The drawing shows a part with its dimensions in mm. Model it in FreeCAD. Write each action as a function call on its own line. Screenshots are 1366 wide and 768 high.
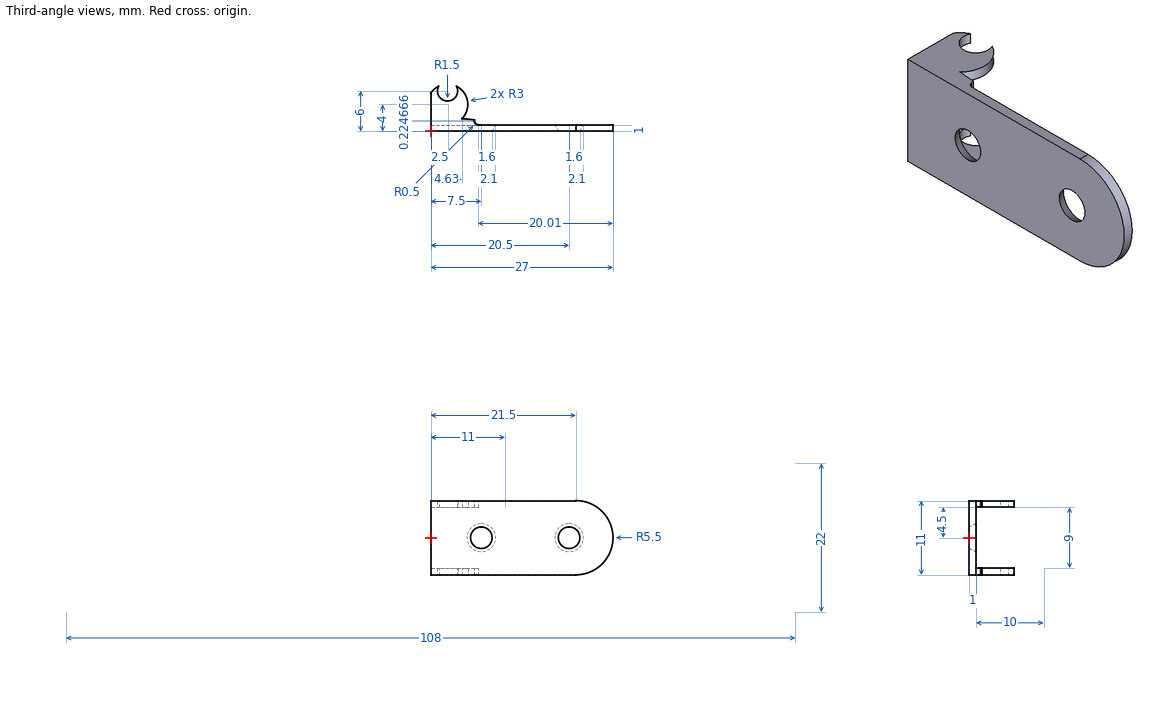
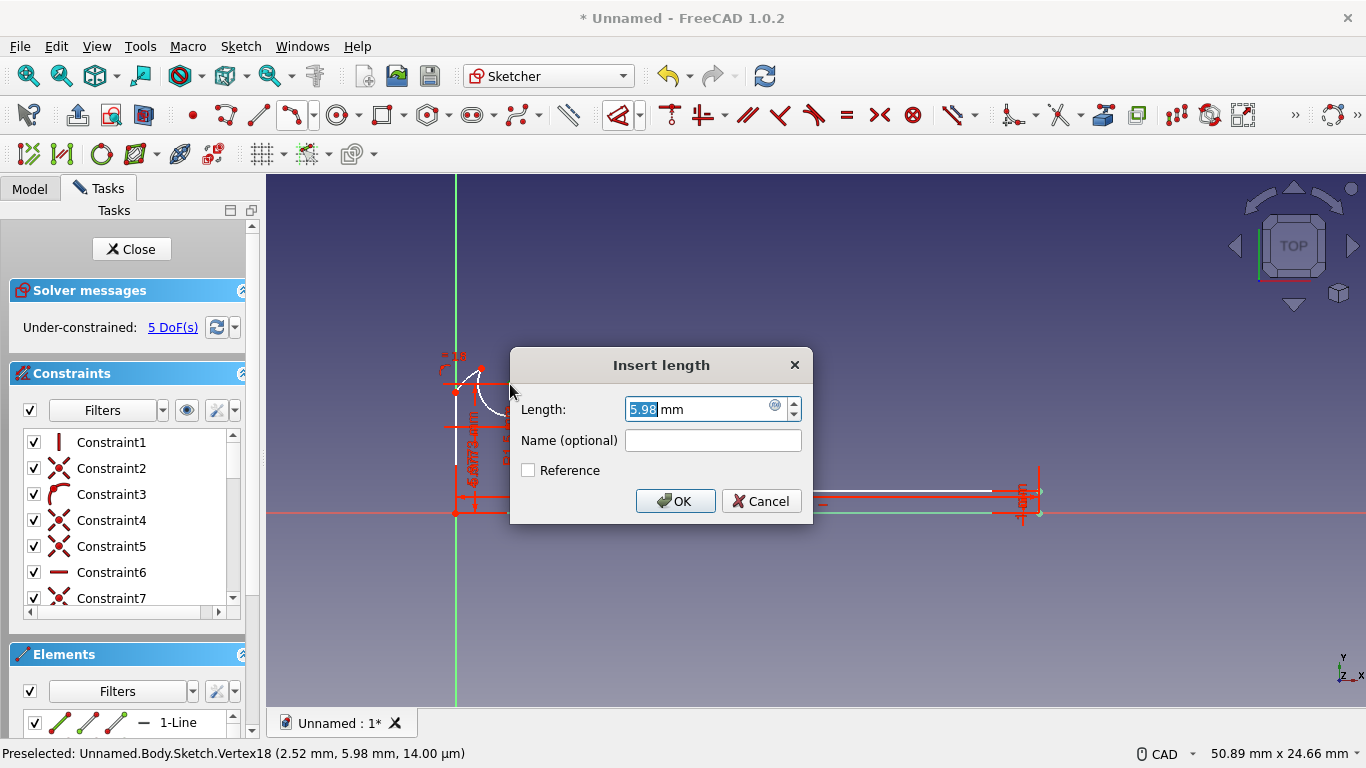
text(6)
key(Return)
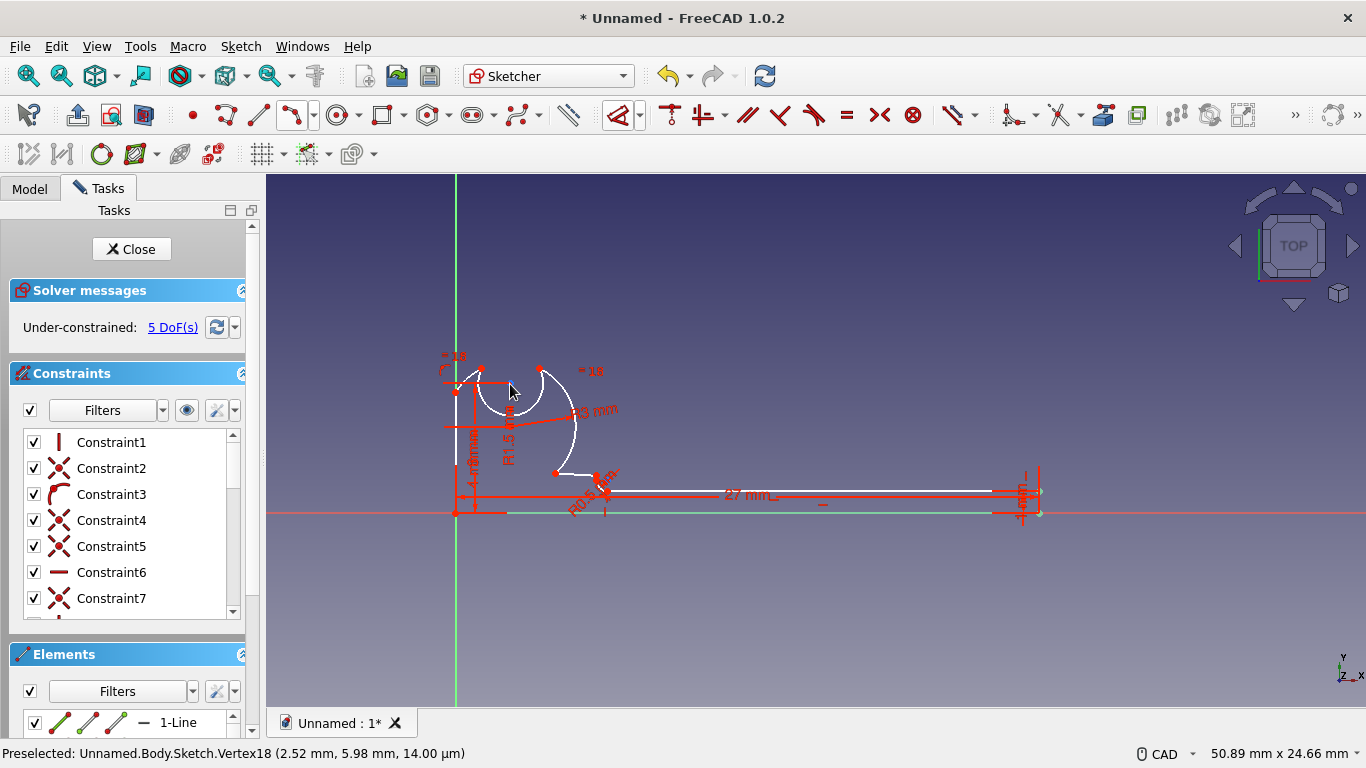
click(511, 427)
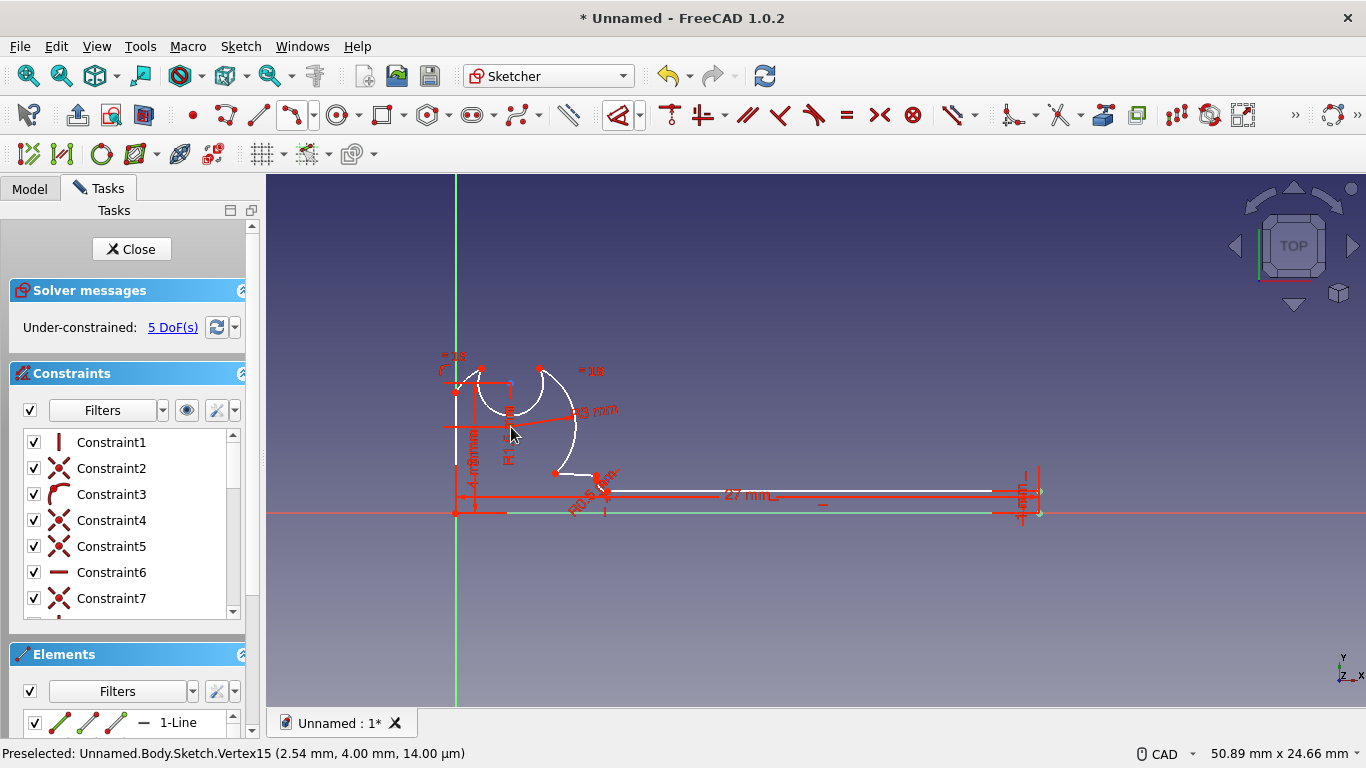
key(l)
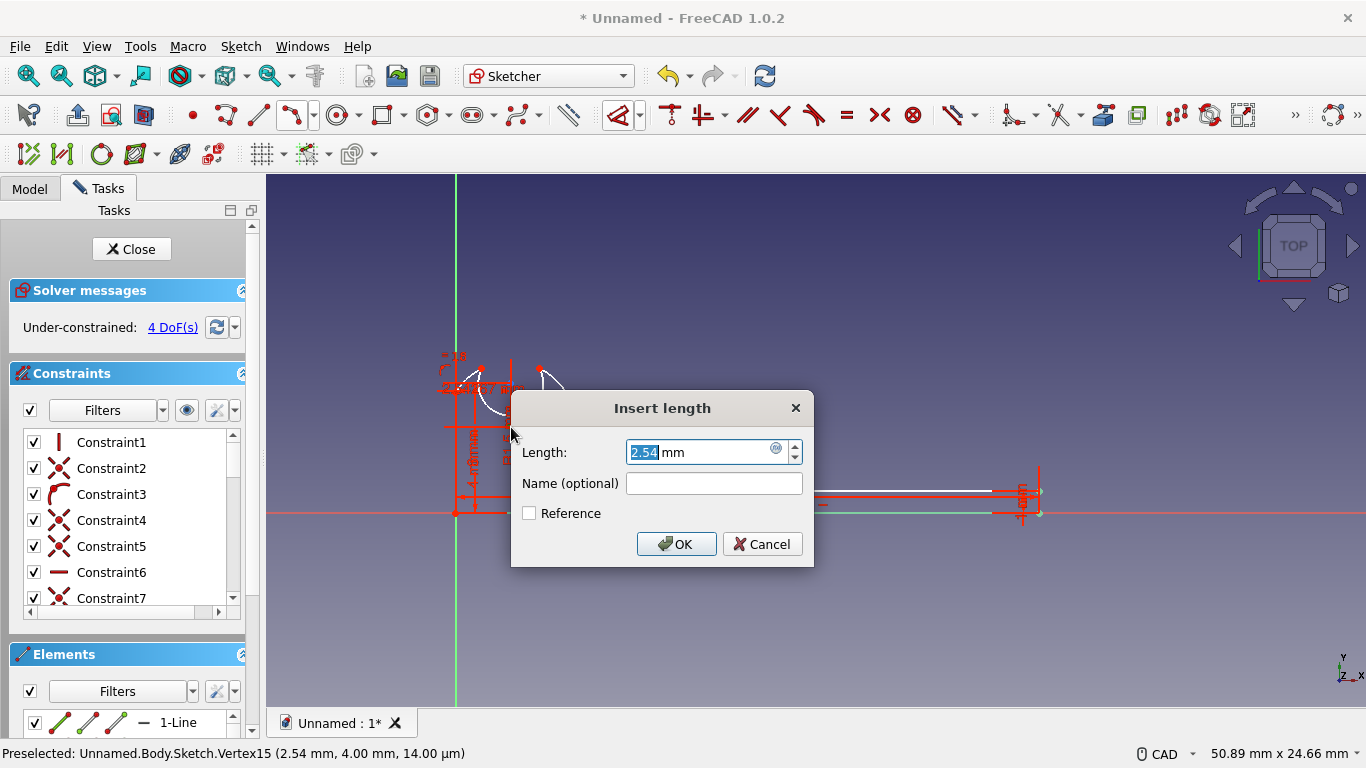
text(2.5)
key(Return)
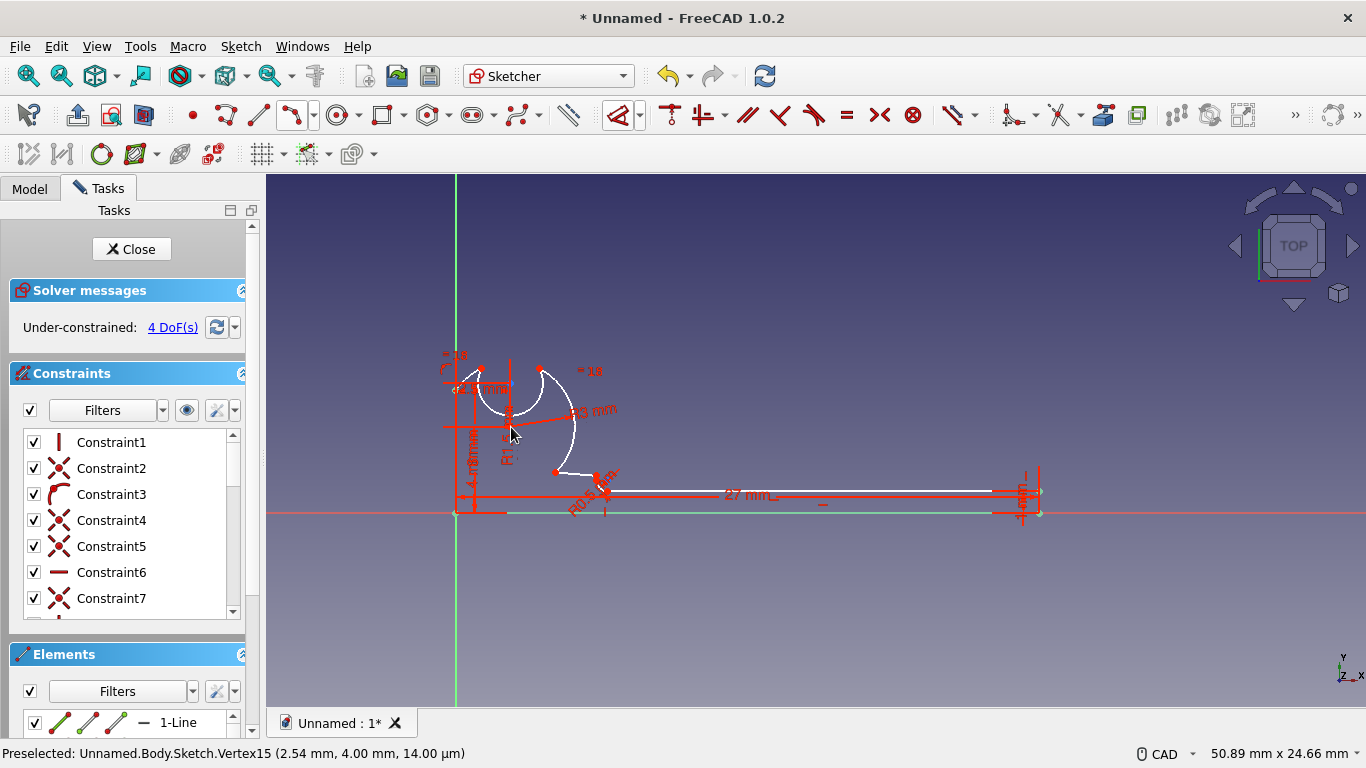
click(510, 383)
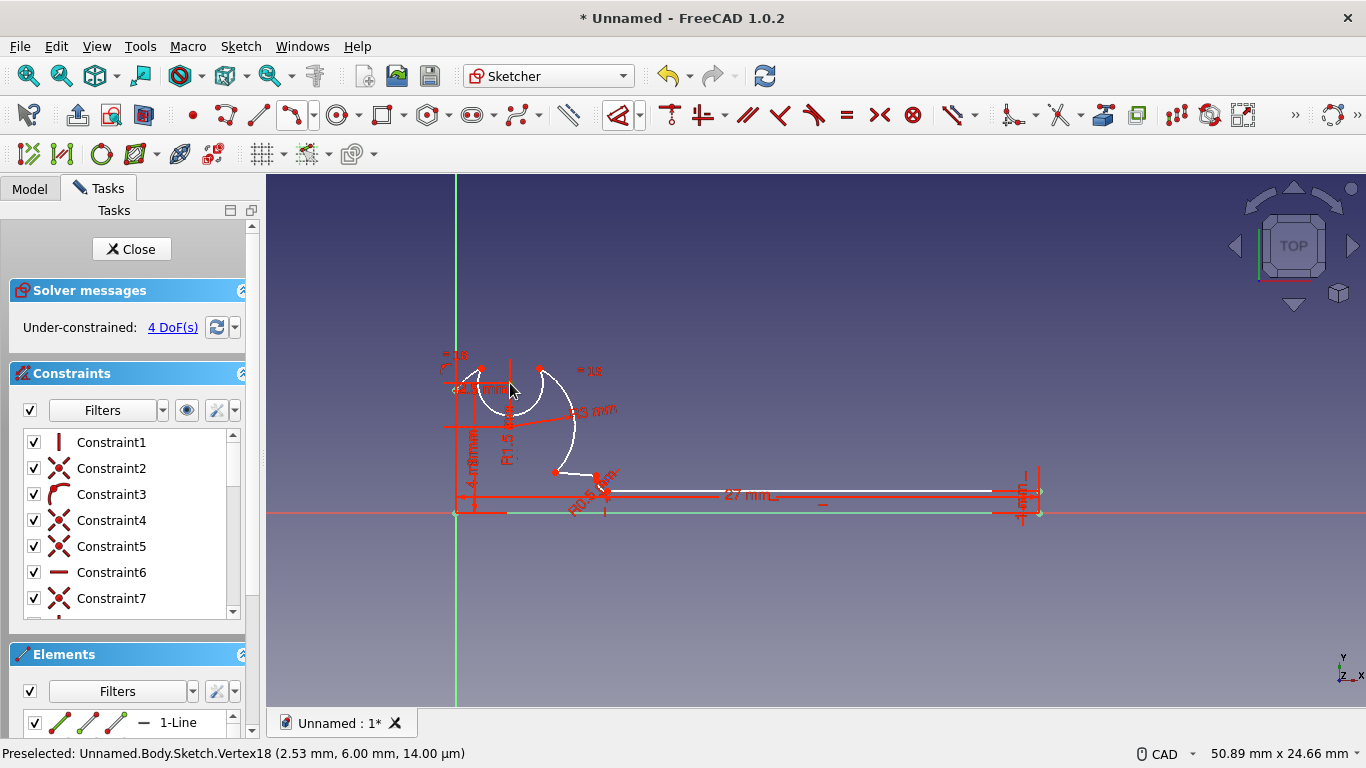
key(l)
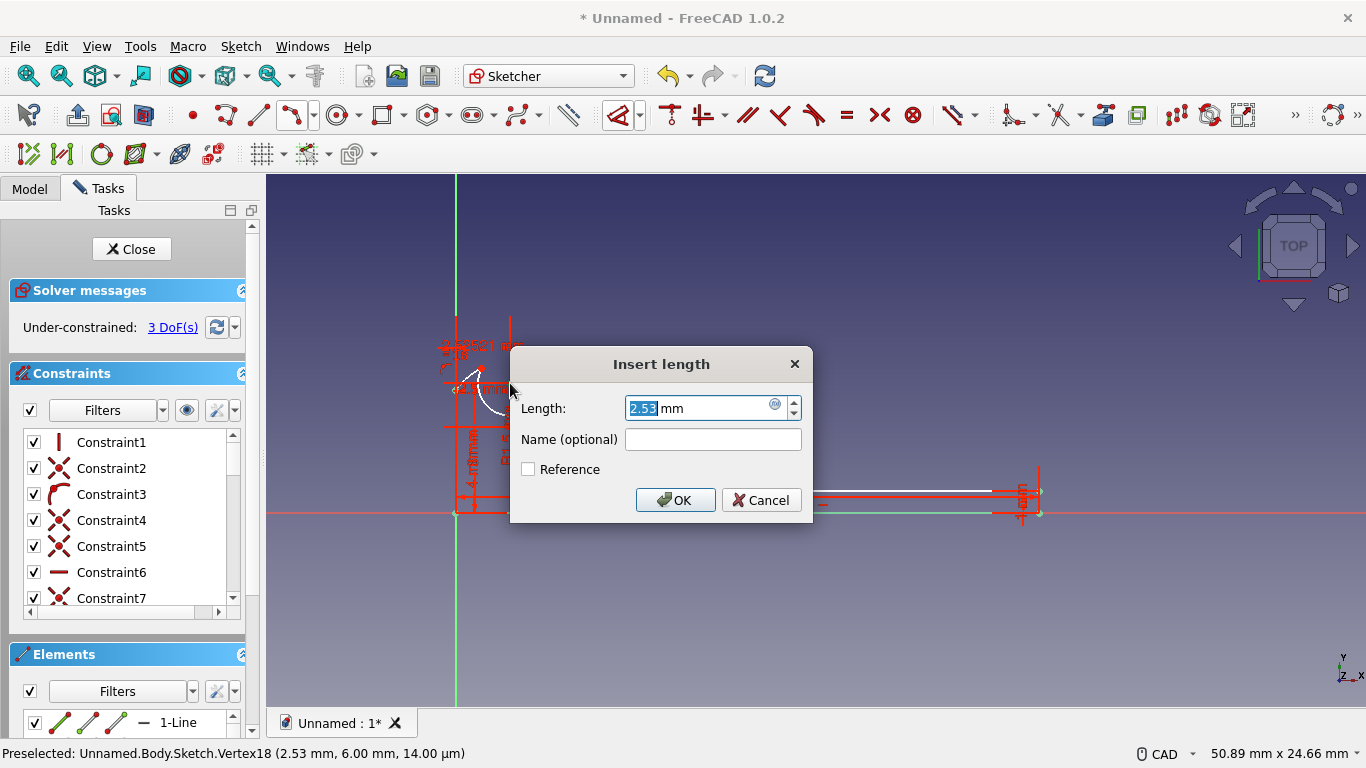
text(2.5)
key(Return)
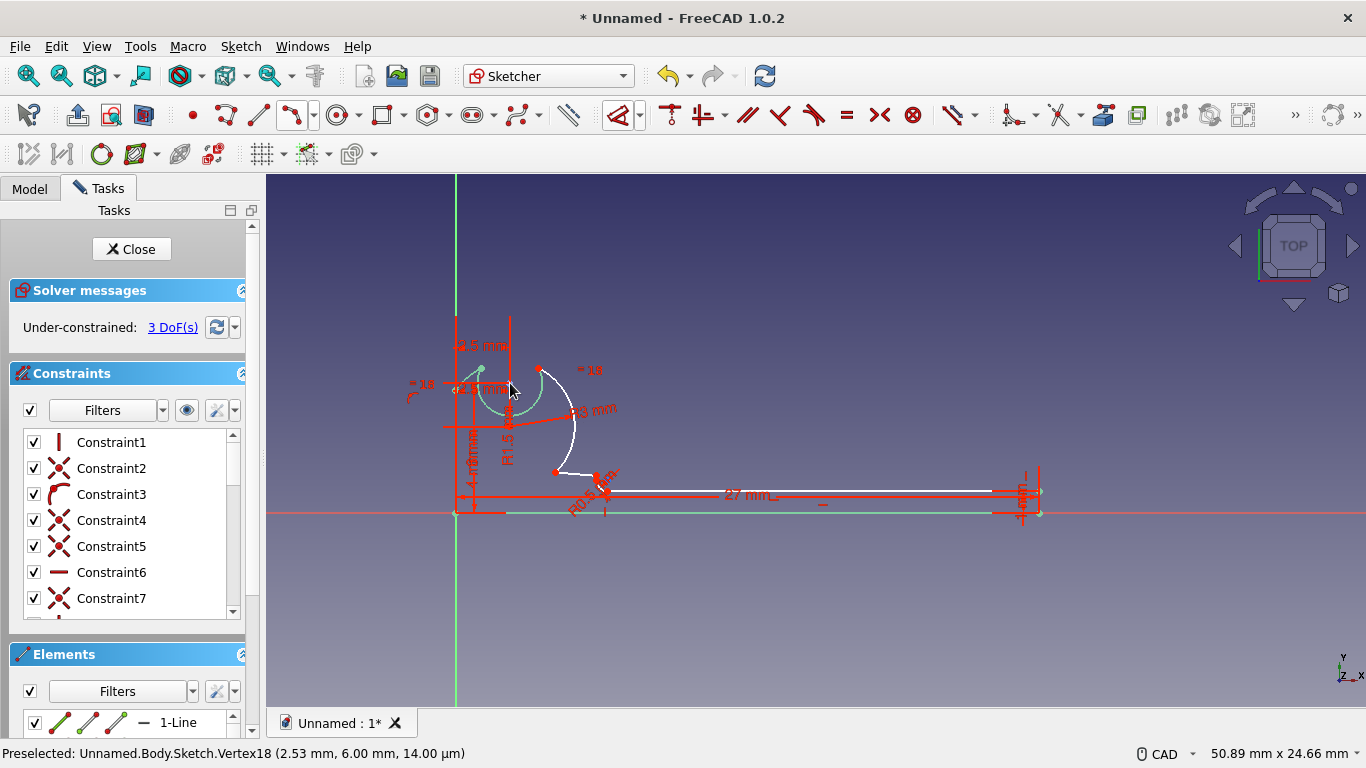
click(910, 491)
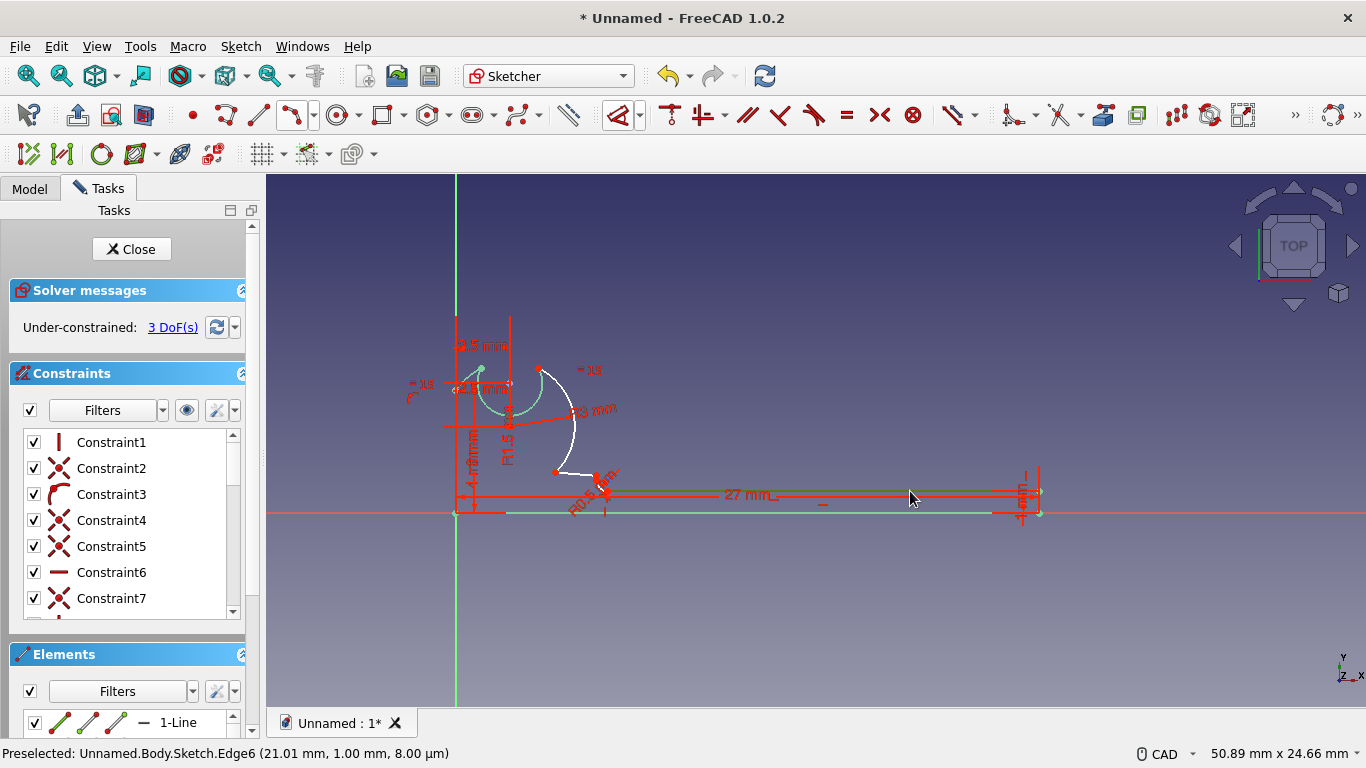
key(l)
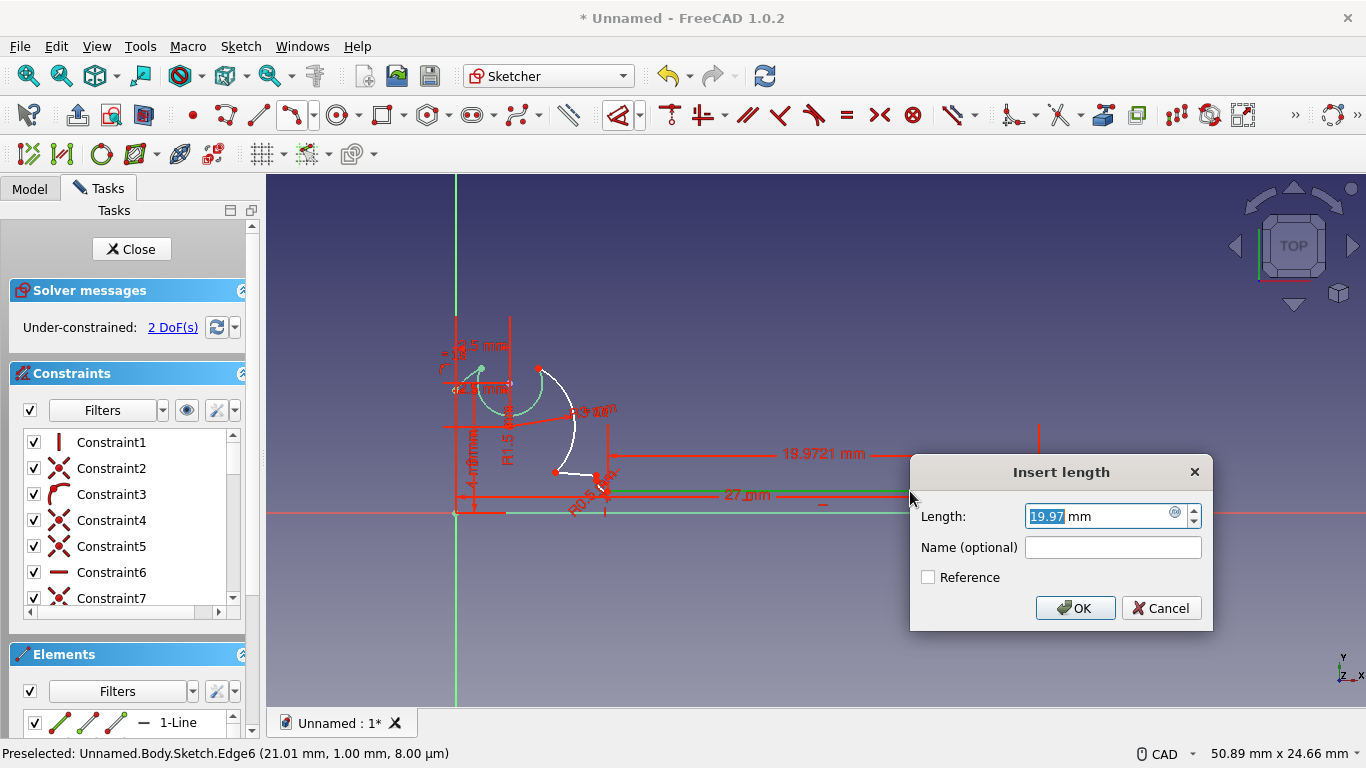
text(20.01)
key(Return)